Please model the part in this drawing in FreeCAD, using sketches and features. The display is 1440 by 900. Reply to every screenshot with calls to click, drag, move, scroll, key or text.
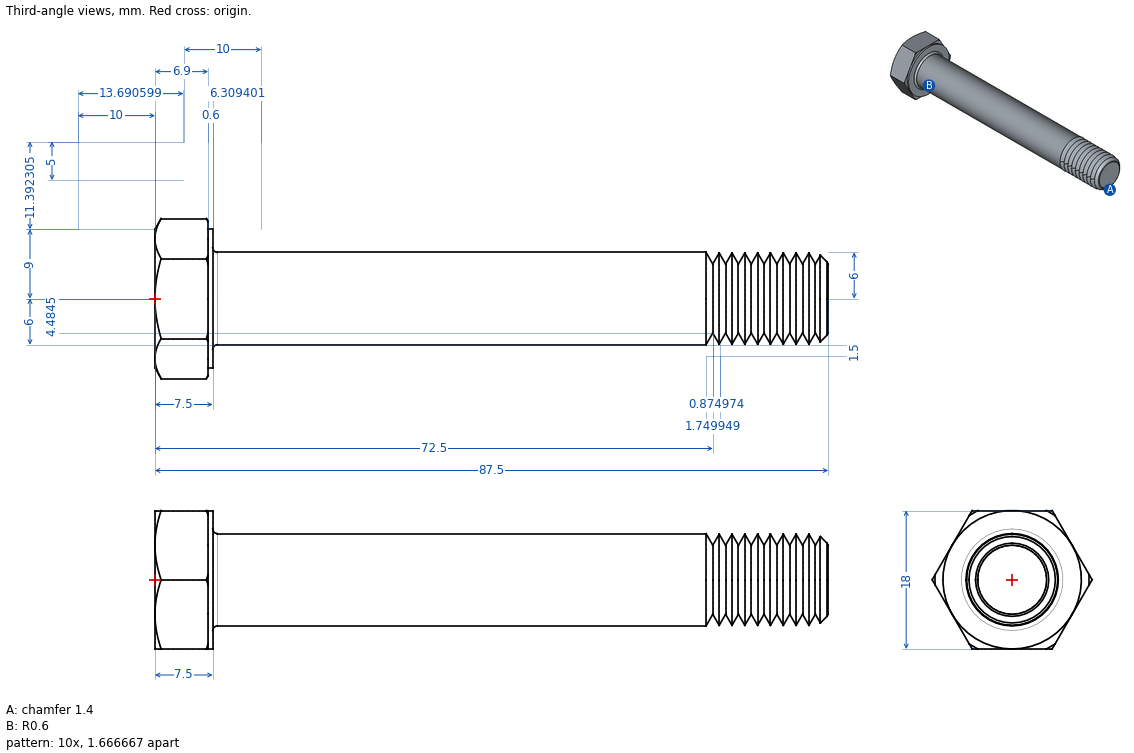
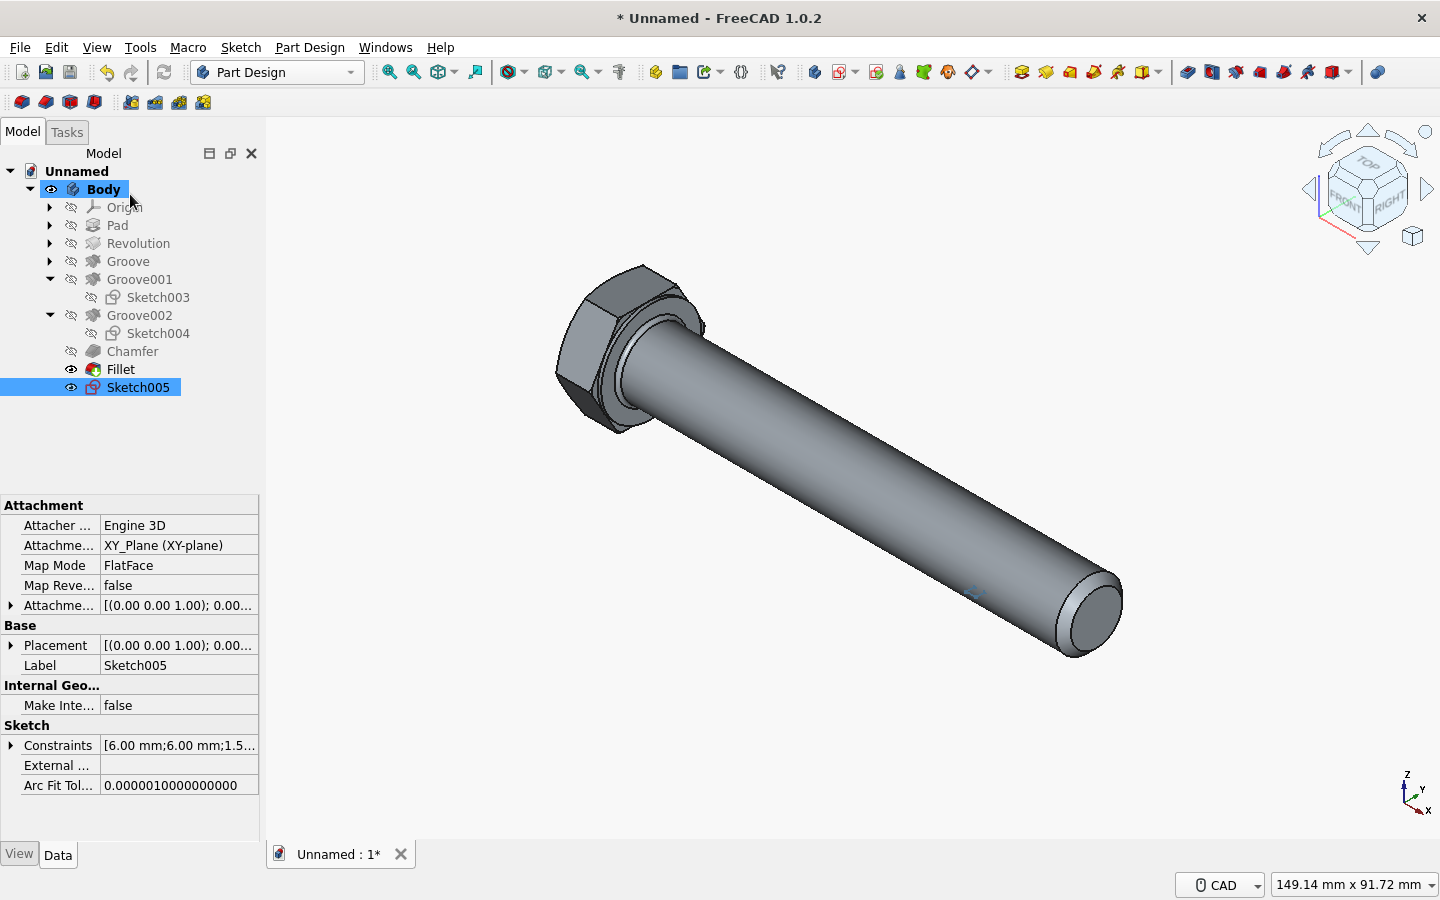
click(1236, 72)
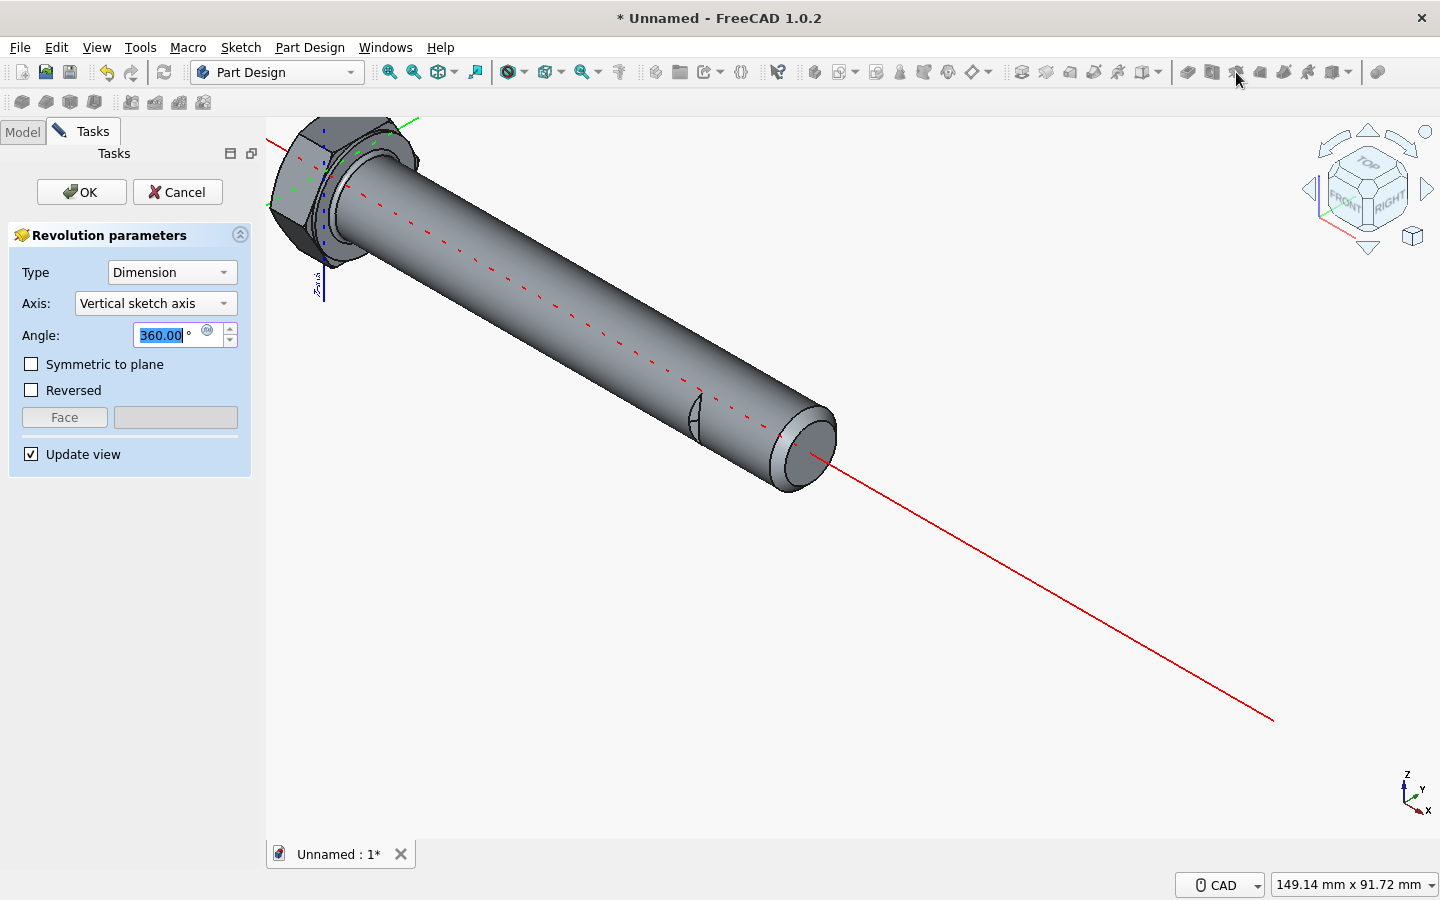
click(156, 304)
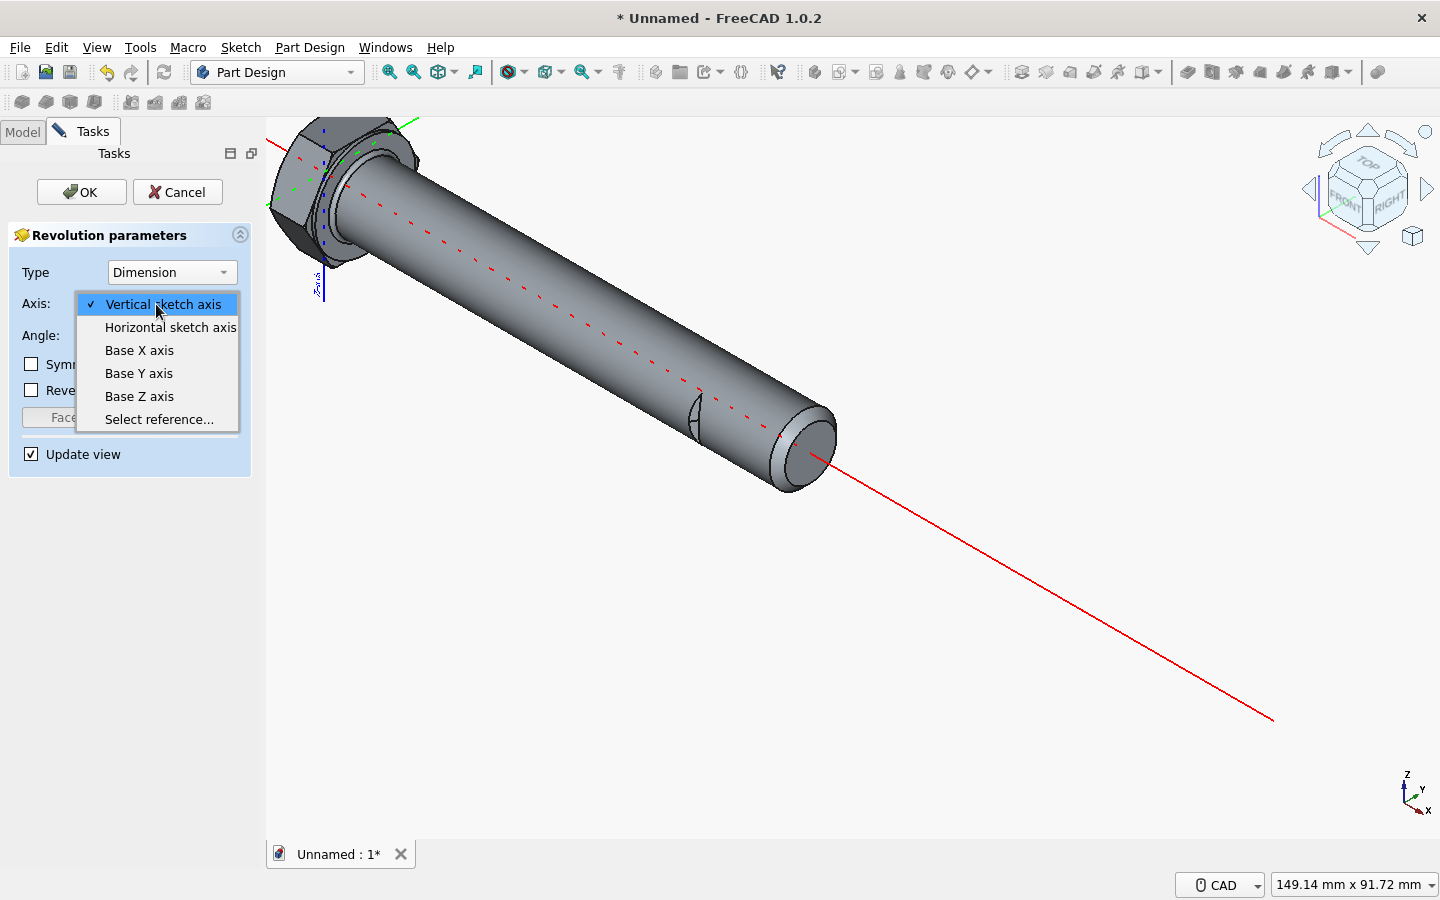
click(156, 328)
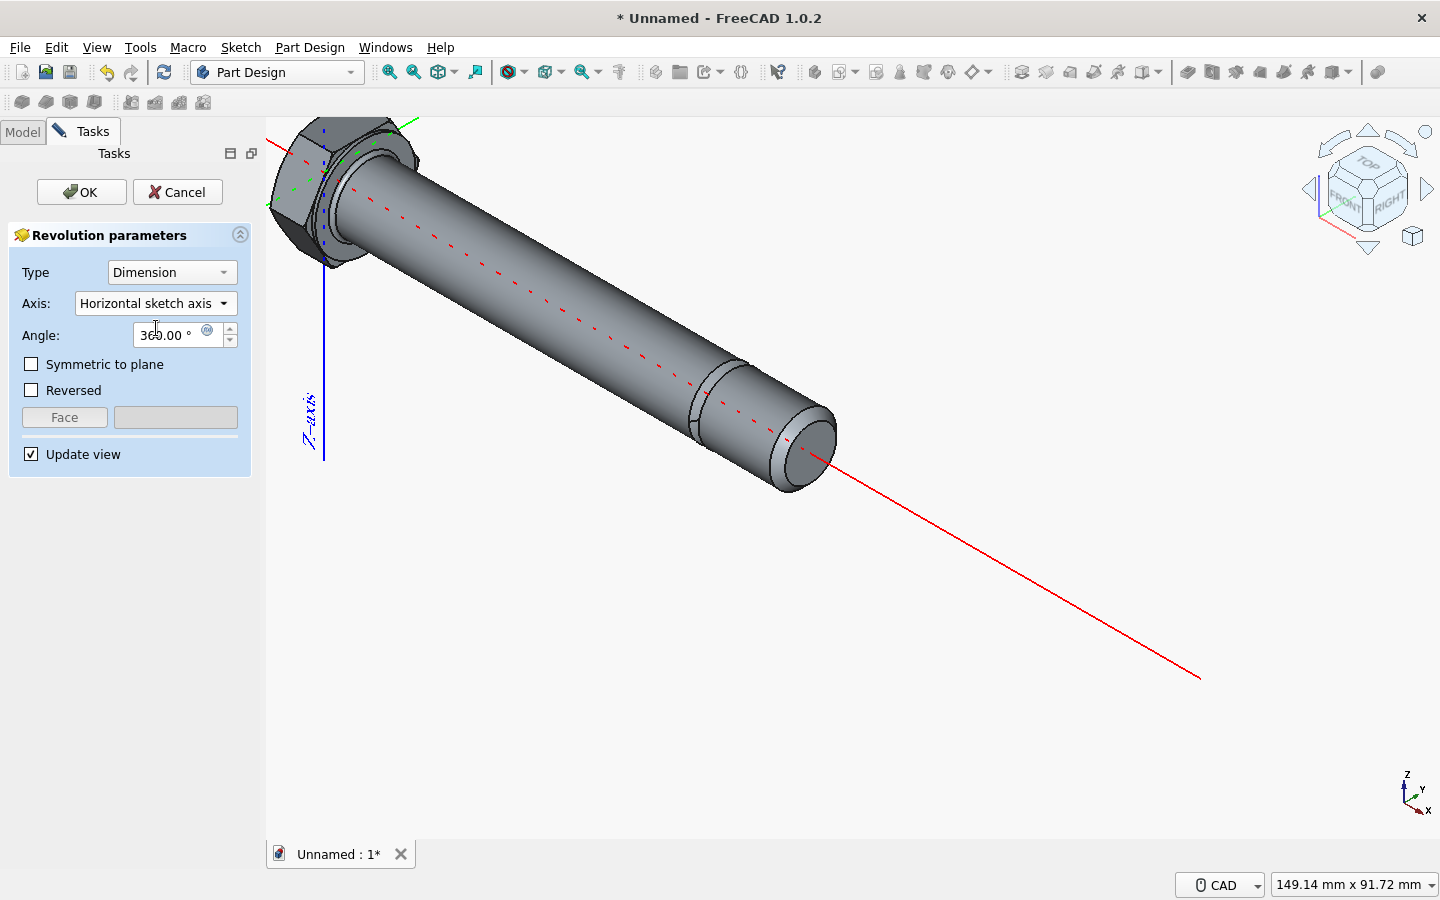
click(82, 192)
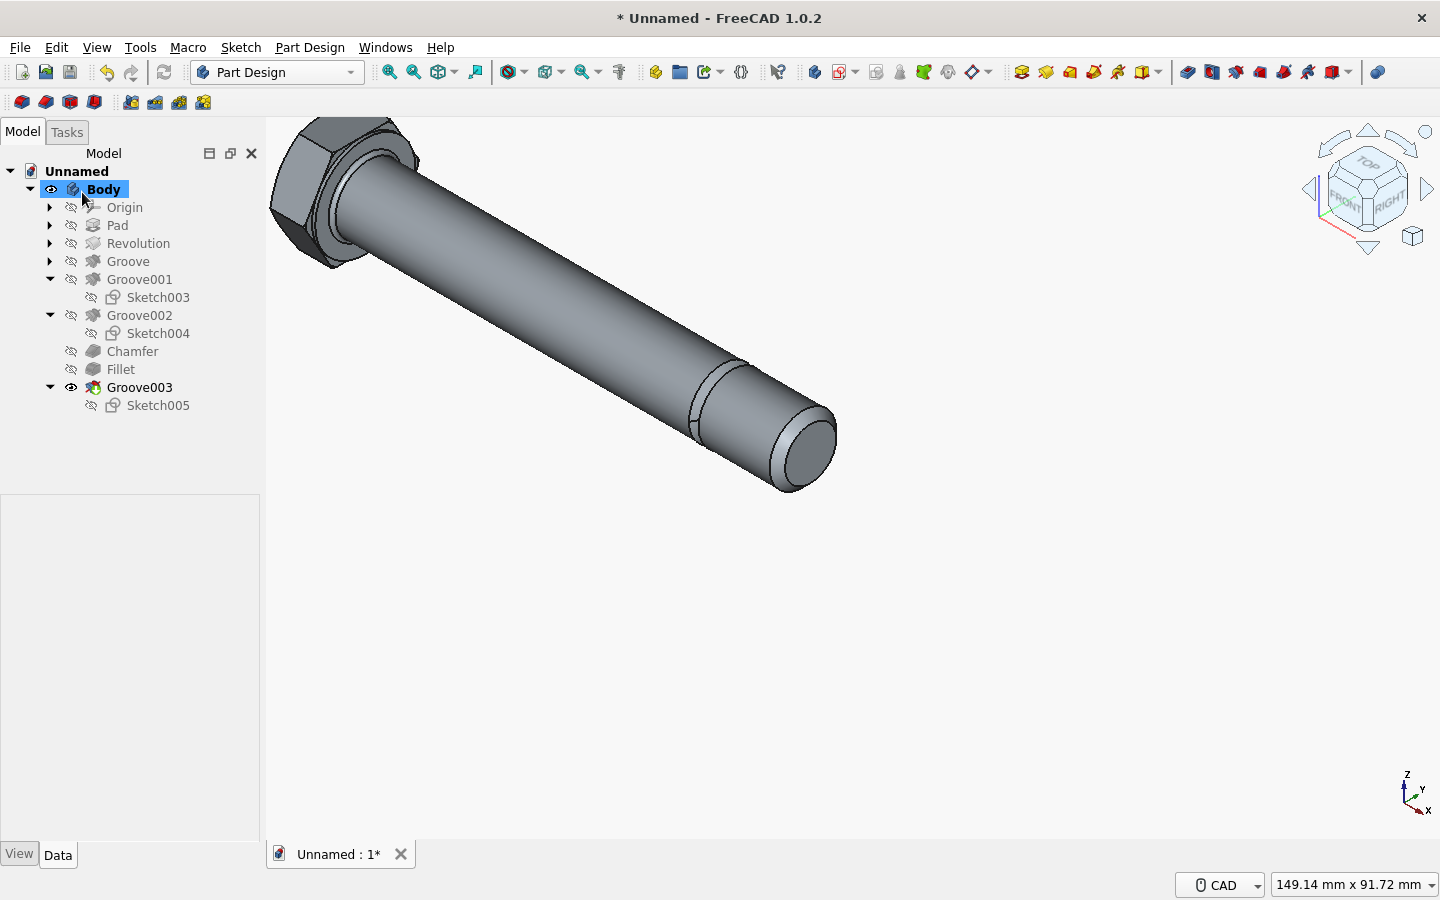
click(390, 72)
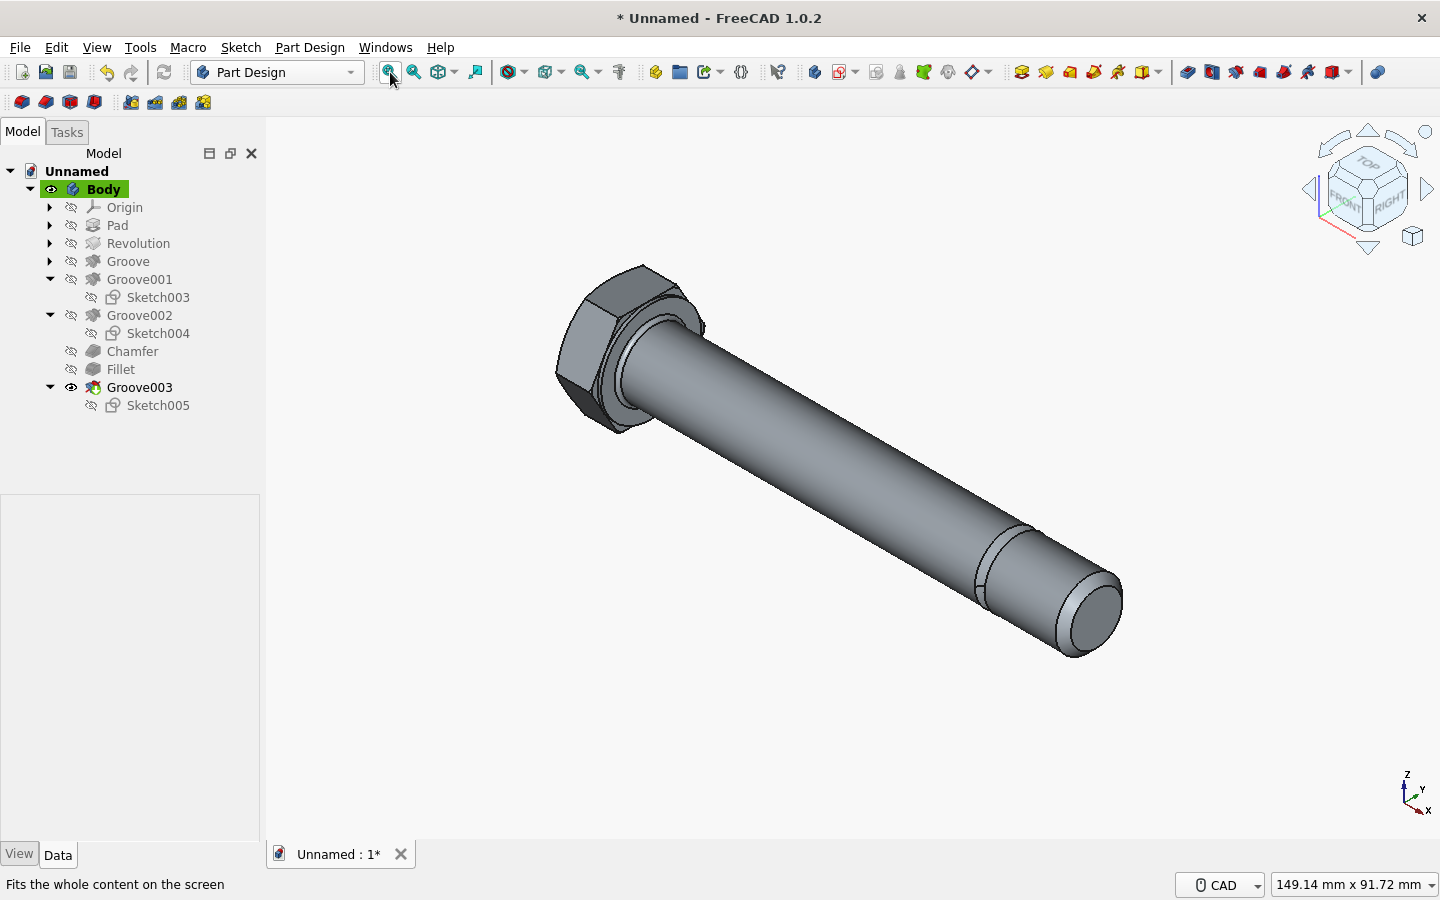
click(116, 387)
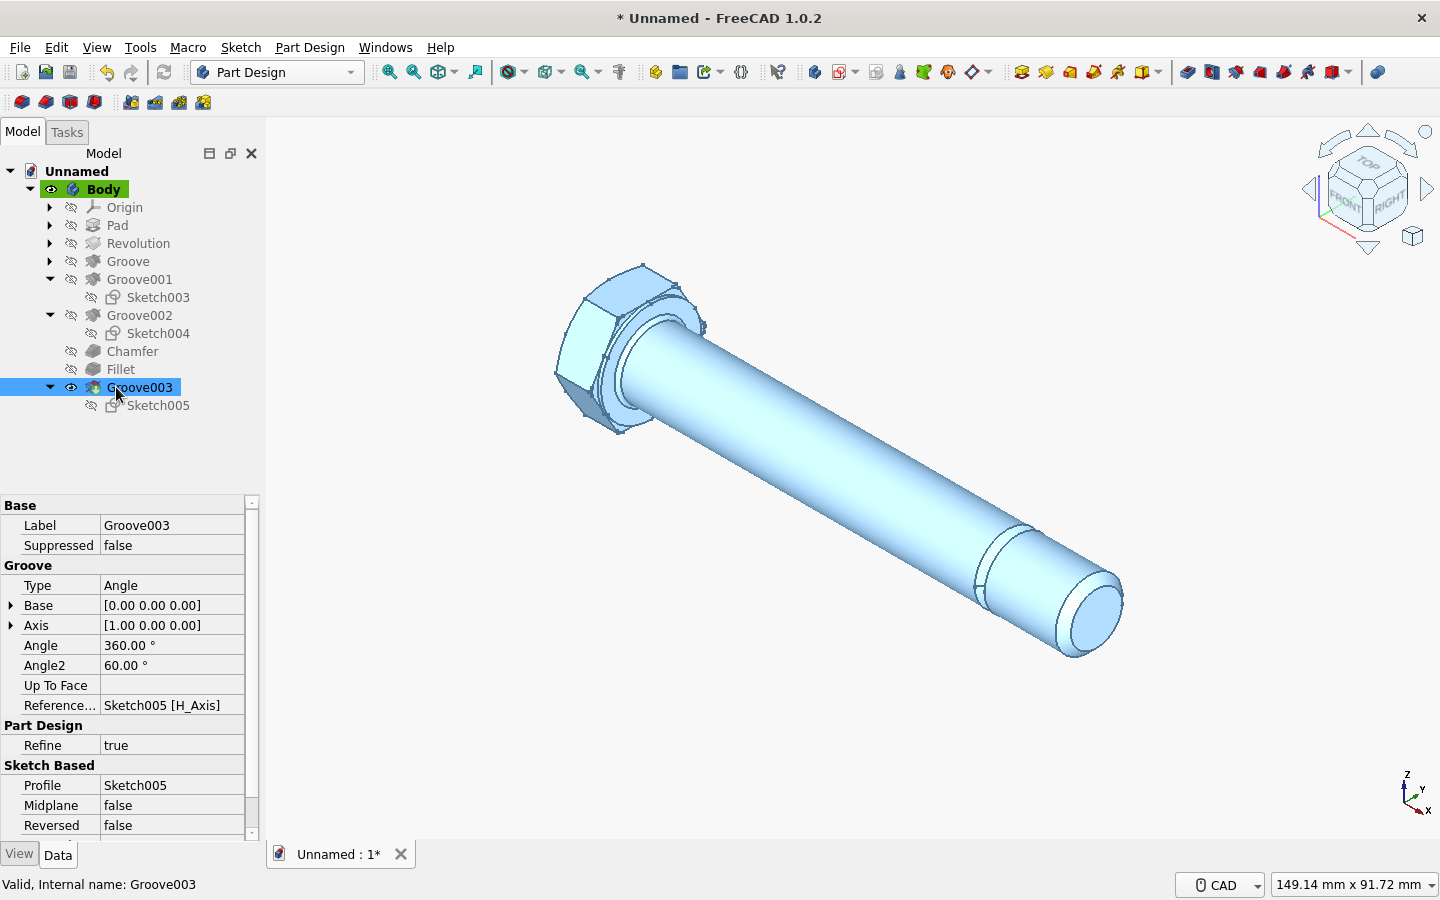
click(156, 102)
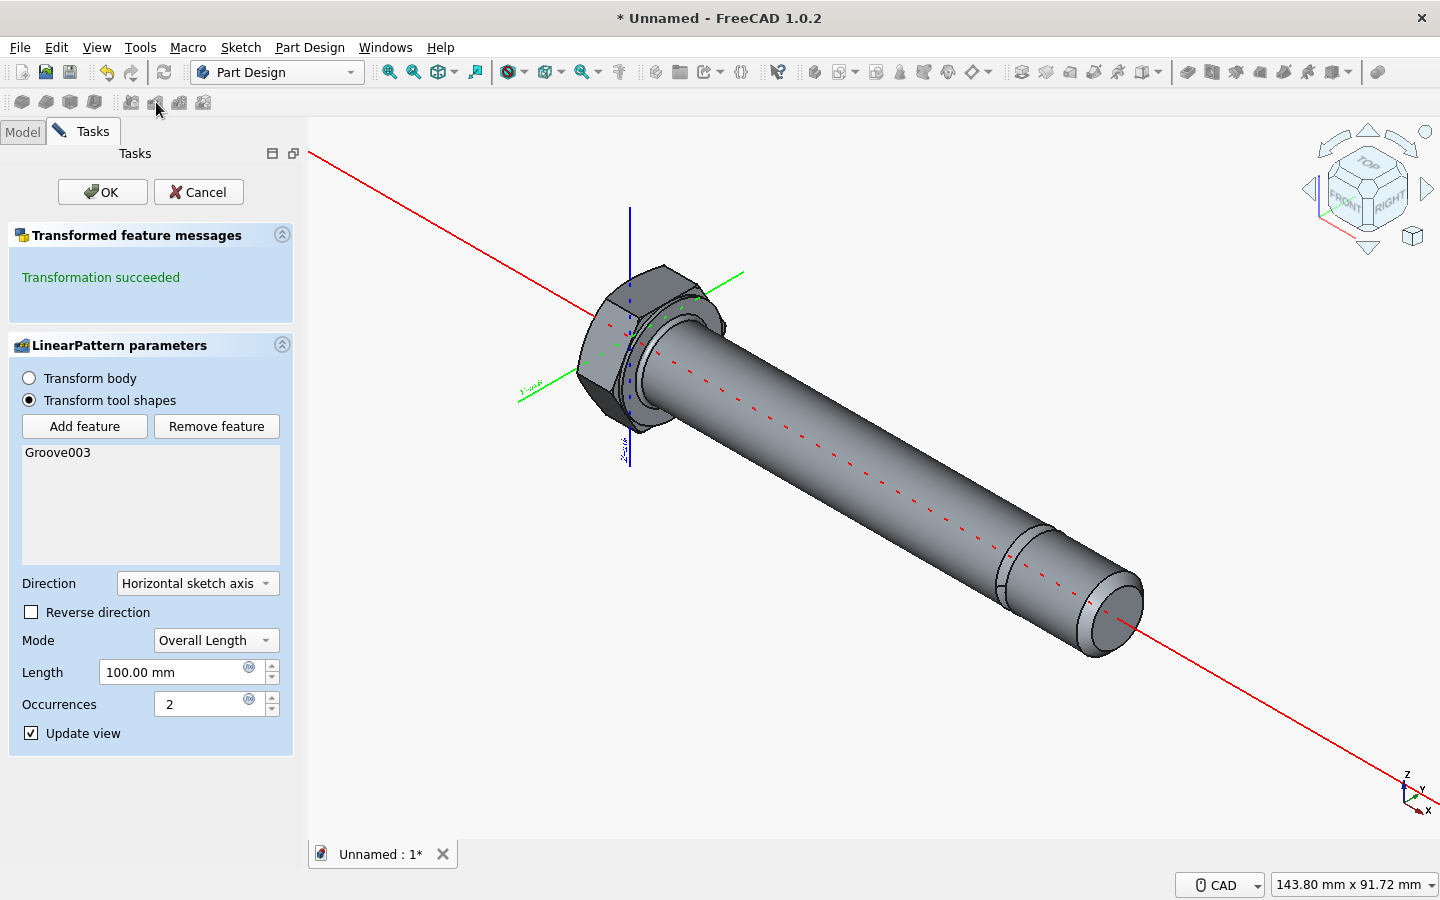
click(198, 584)